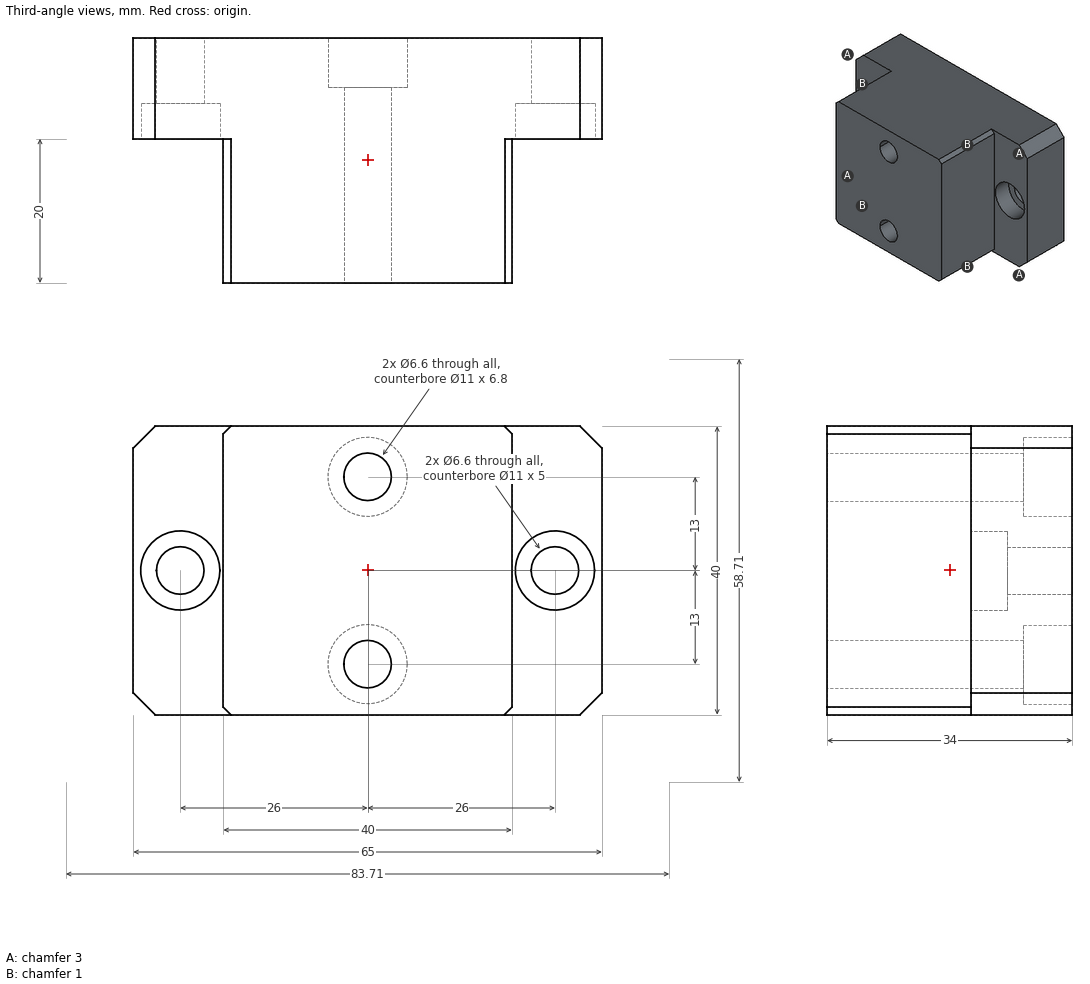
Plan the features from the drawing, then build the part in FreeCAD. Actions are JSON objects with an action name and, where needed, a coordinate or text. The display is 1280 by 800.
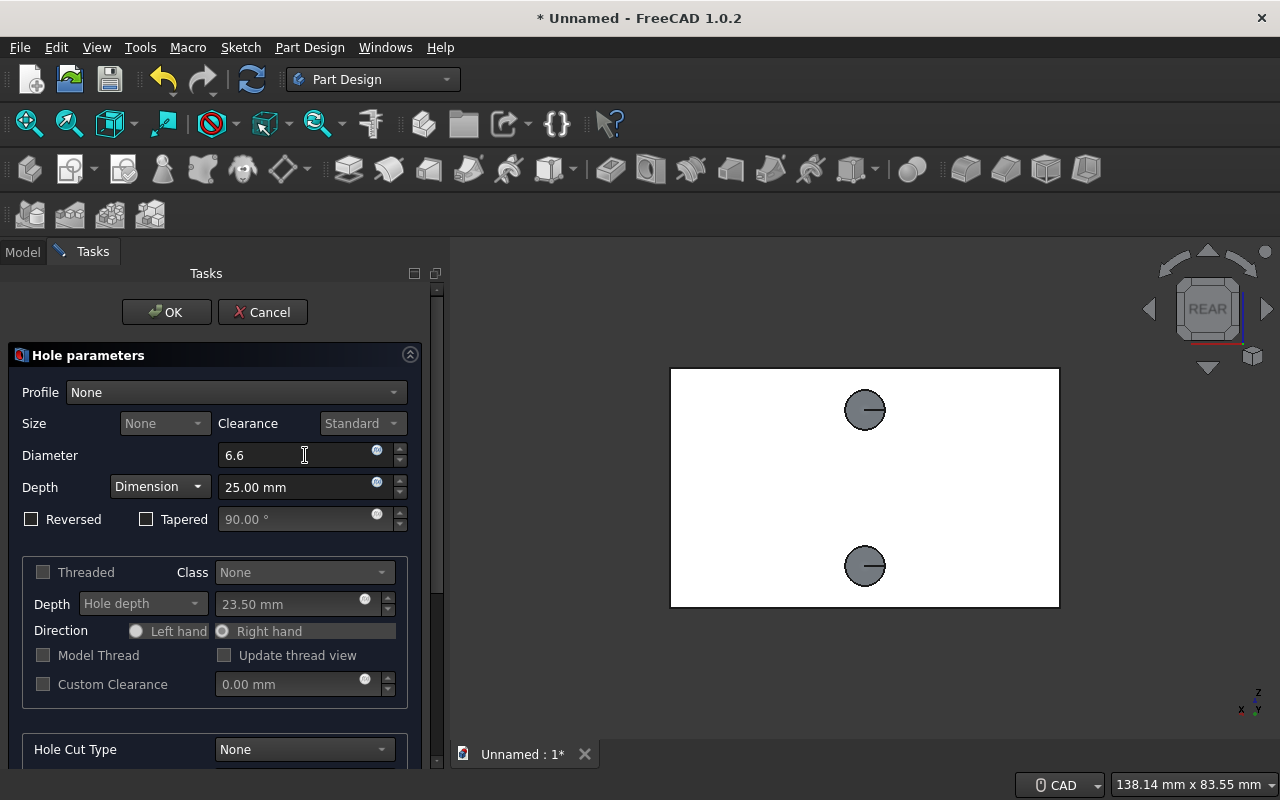
{"action": "left_click", "coordinate": [161, 486]}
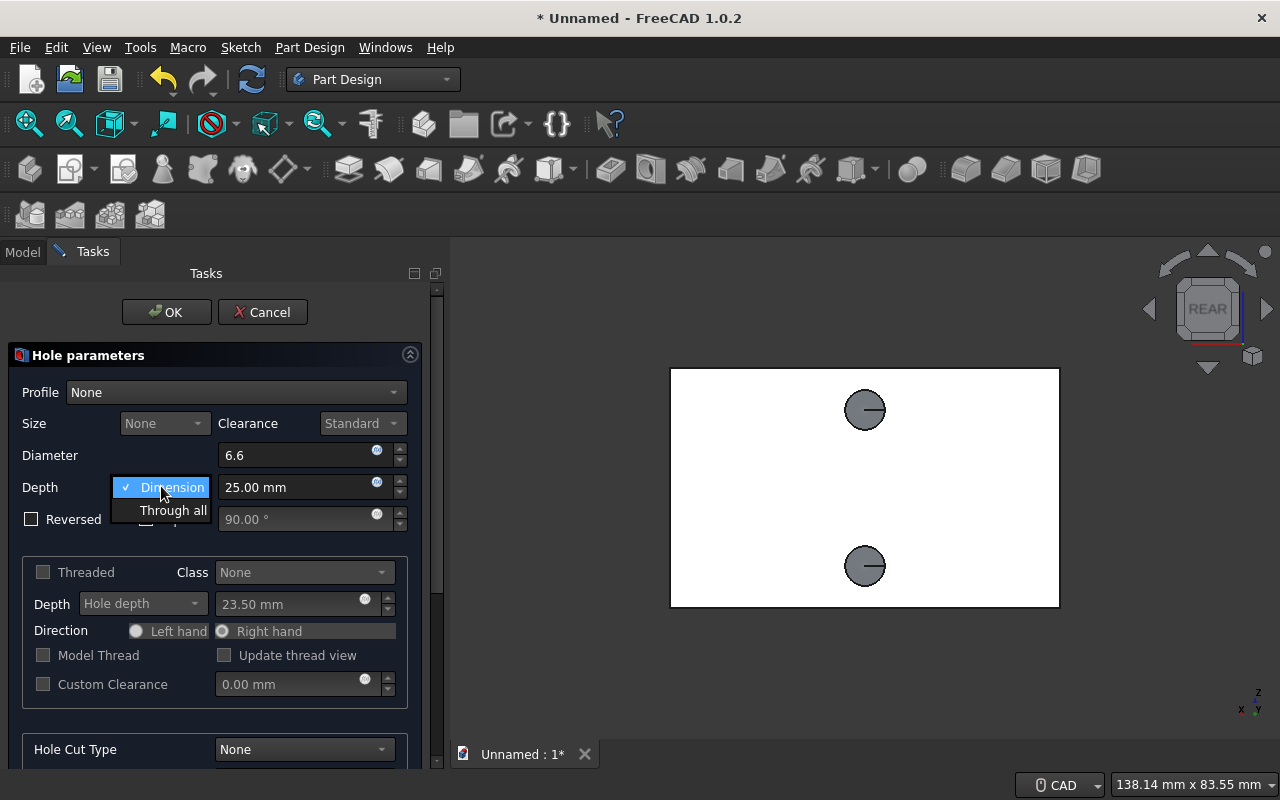
{"action": "left_click", "coordinate": [160, 510]}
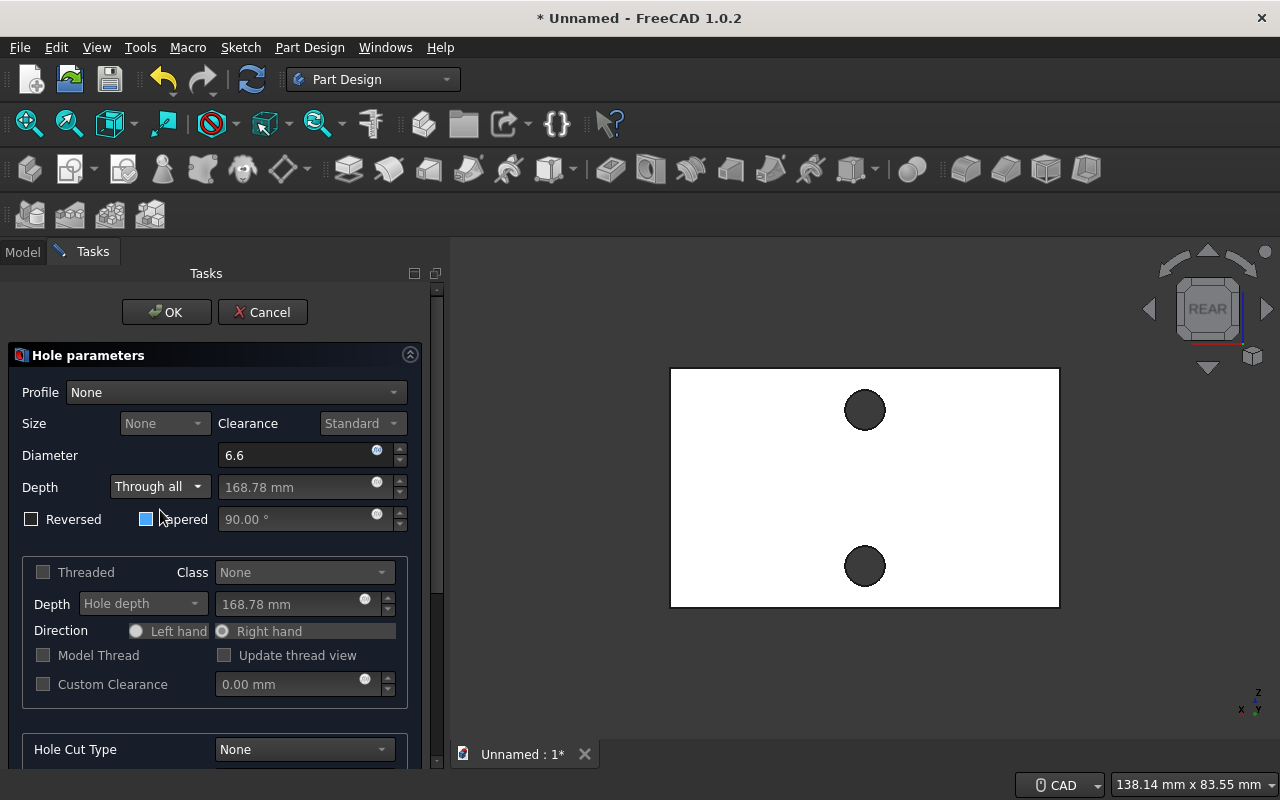
{"action": "left_click", "coordinate": [306, 750]}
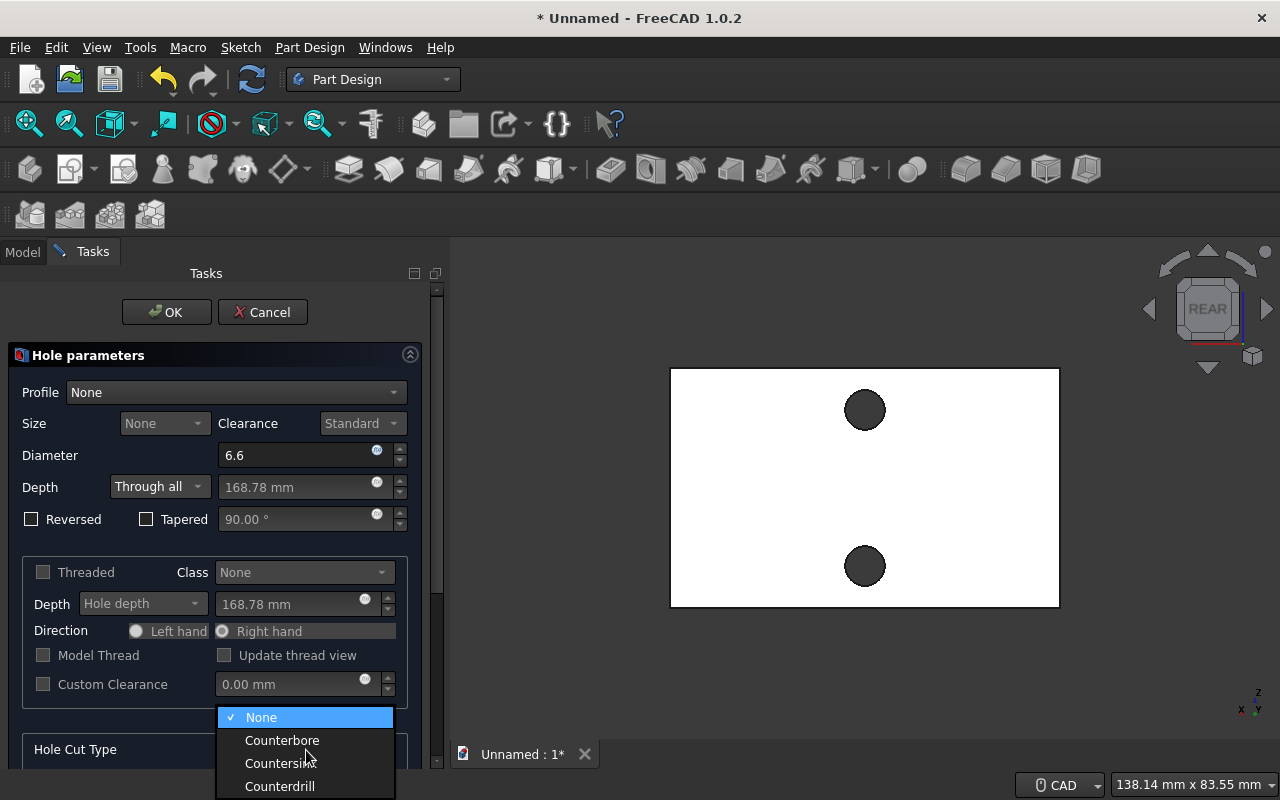
{"action": "left_click", "coordinate": [304, 740]}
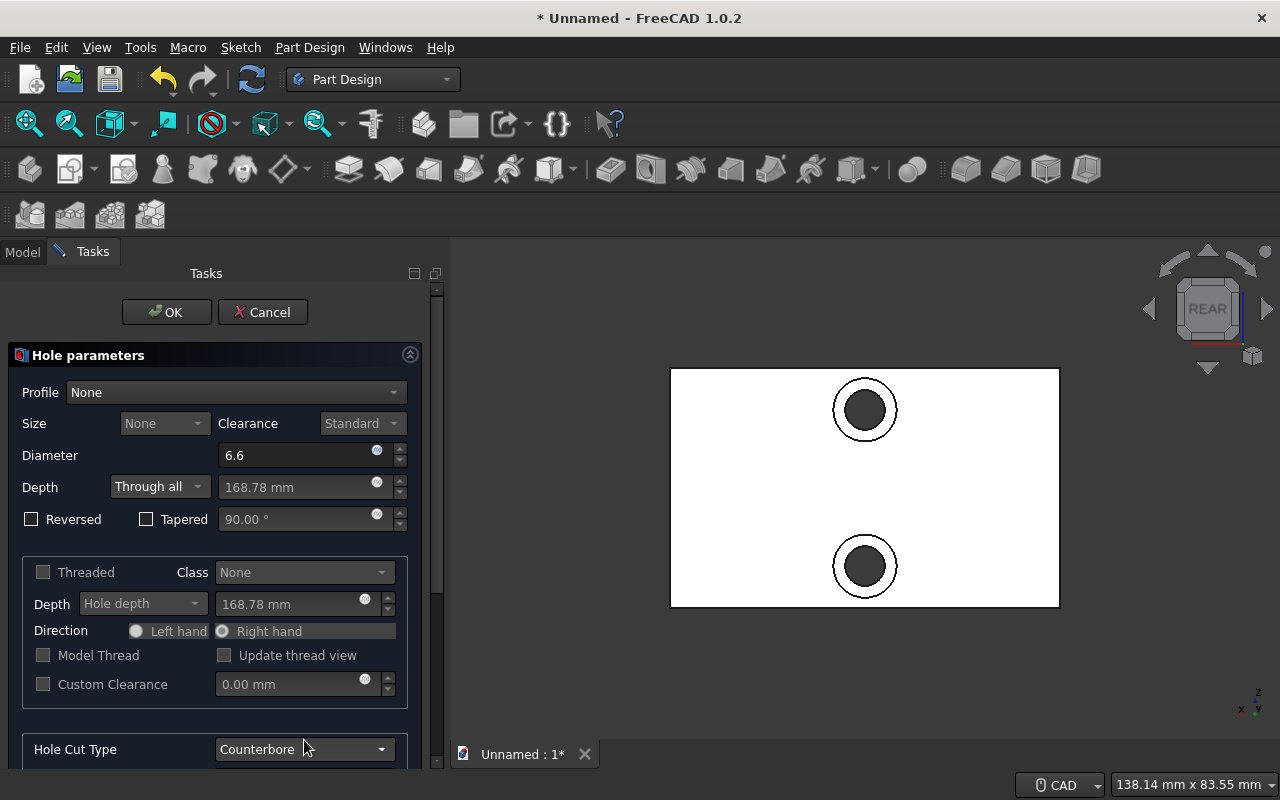
{"action": "scroll", "coordinate": [437, 526], "scroll_direction": "down", "scroll_amount": 2}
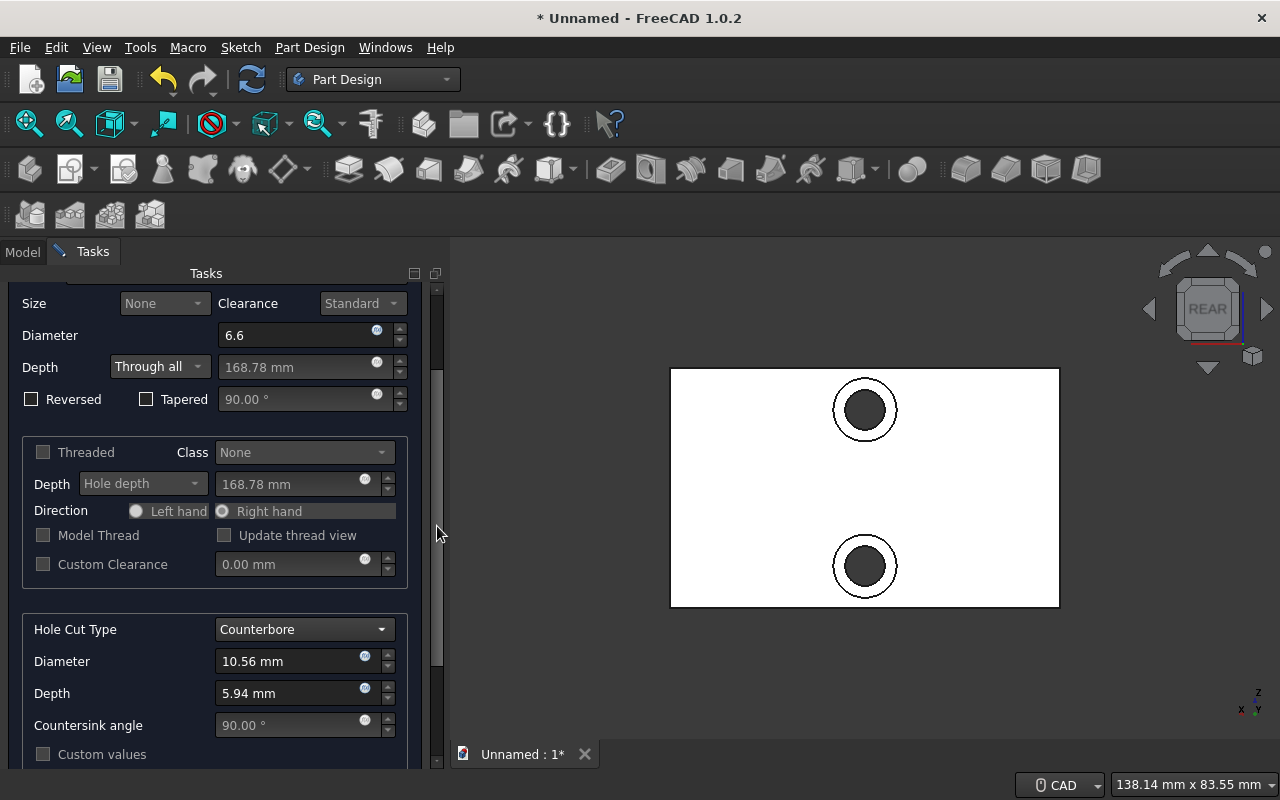
{"action": "triple_click", "coordinate": [298, 661]}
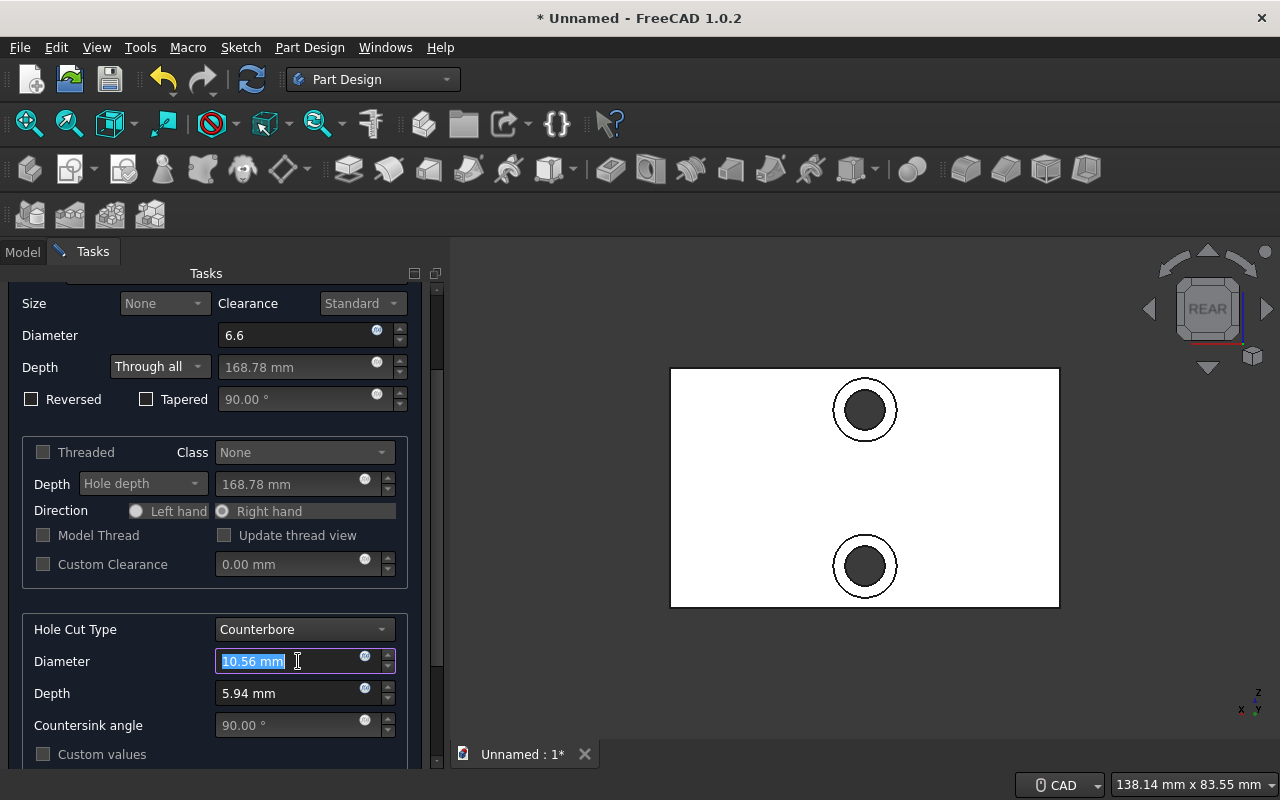
{"action": "type", "text": "11"}
{"action": "key", "text": "Tab"}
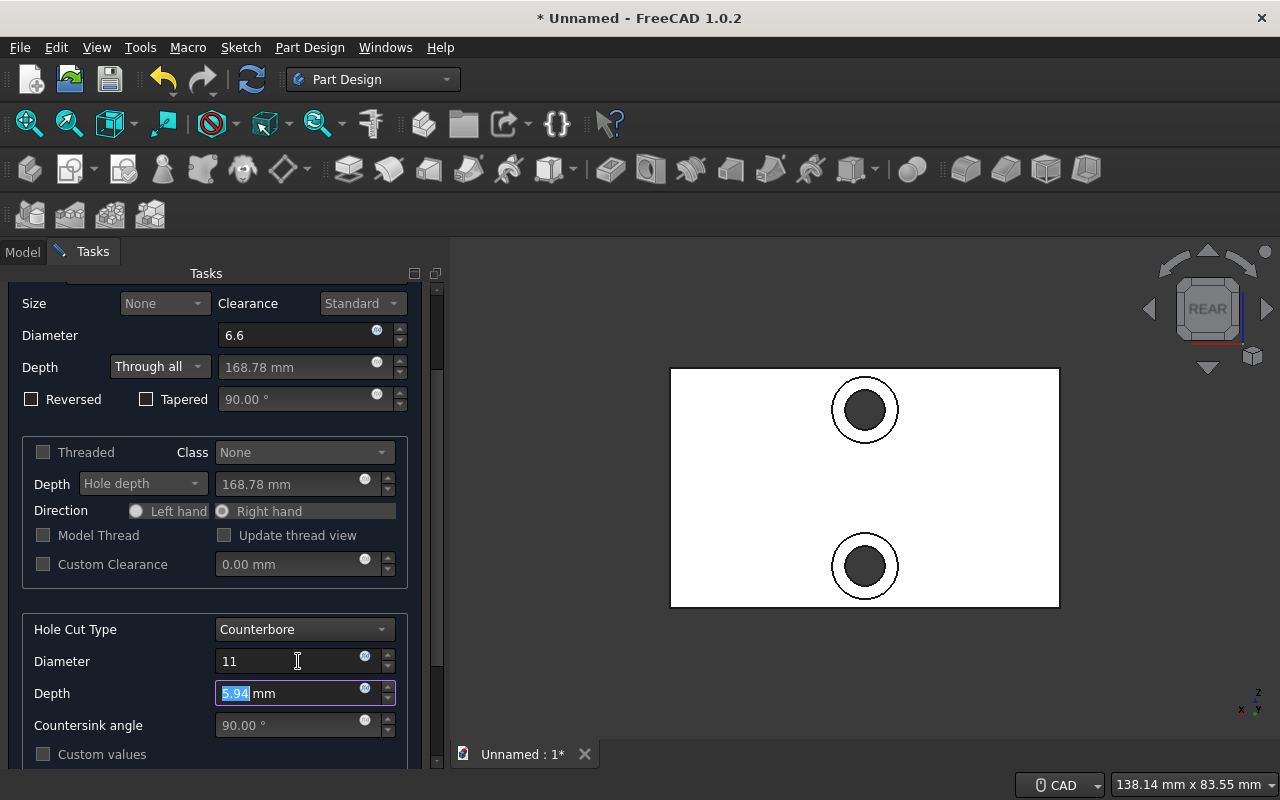
{"action": "type", "text": "6.8"}
{"action": "key", "text": "Tab"}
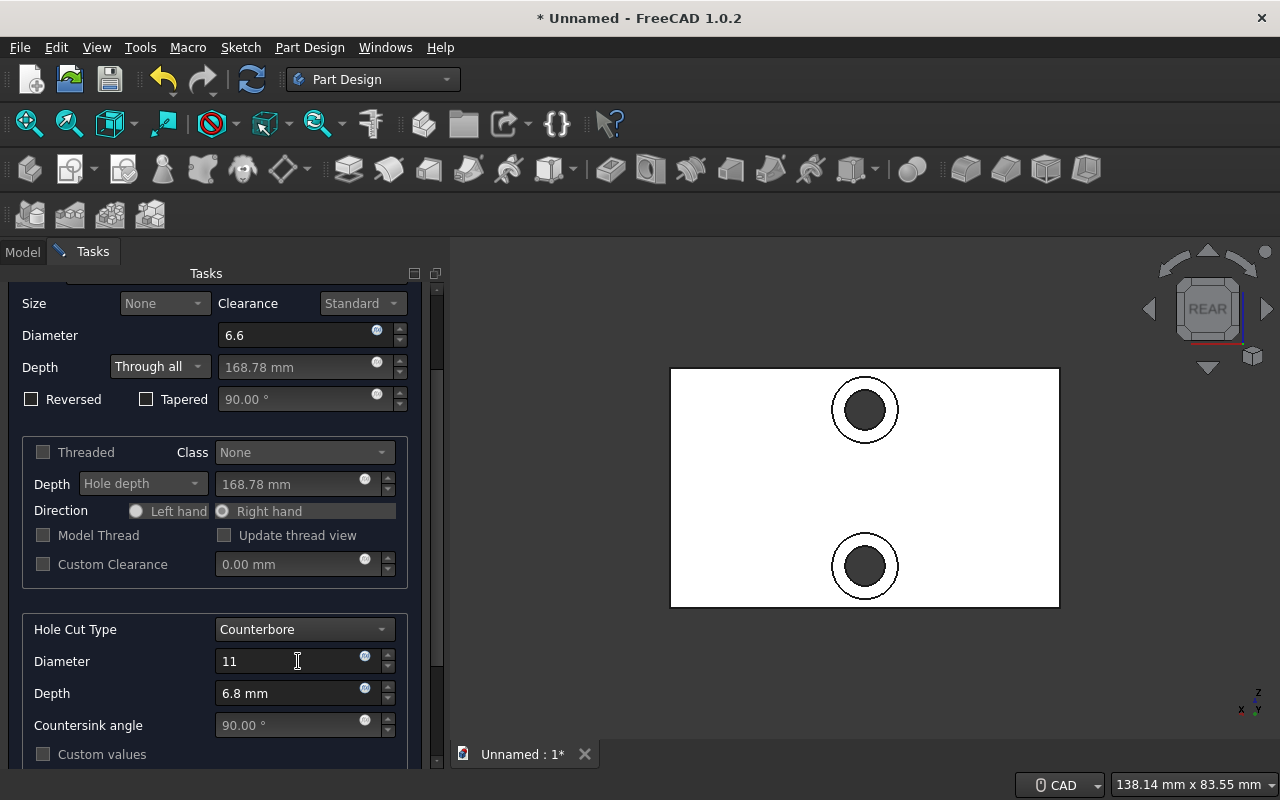
{"action": "scroll", "coordinate": [437, 526], "scroll_direction": "up", "scroll_amount": 3}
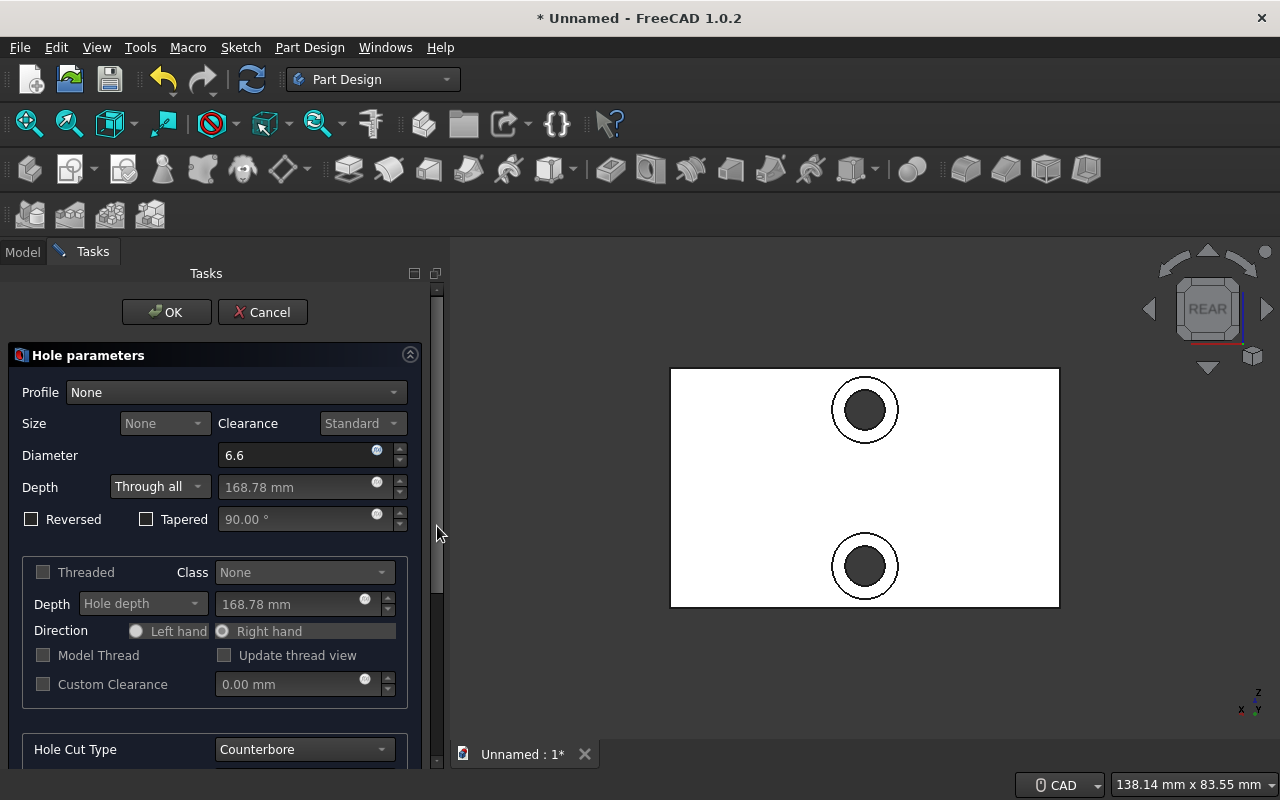
{"action": "left_click", "coordinate": [167, 312]}